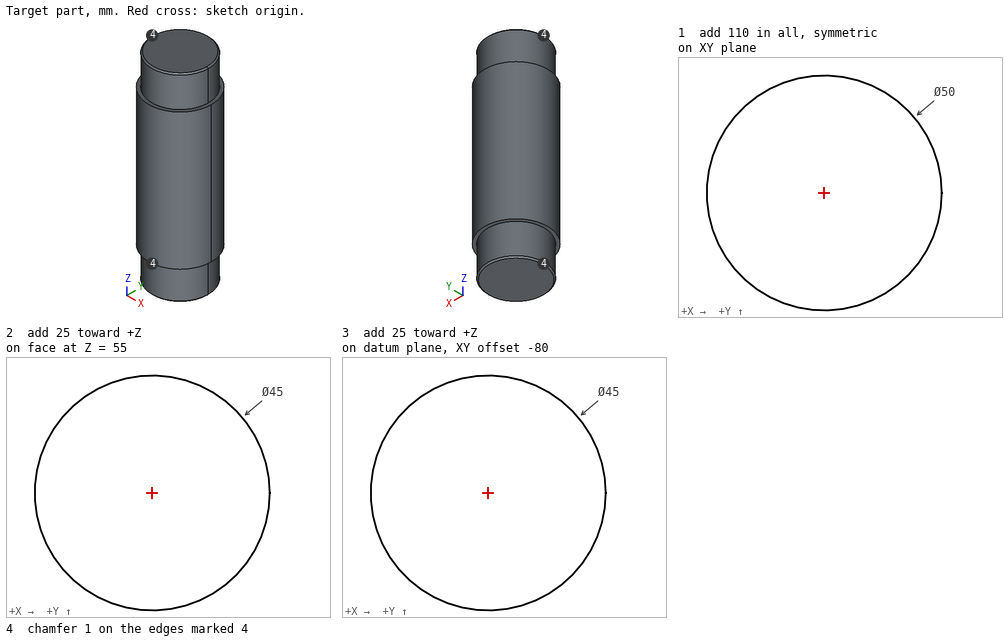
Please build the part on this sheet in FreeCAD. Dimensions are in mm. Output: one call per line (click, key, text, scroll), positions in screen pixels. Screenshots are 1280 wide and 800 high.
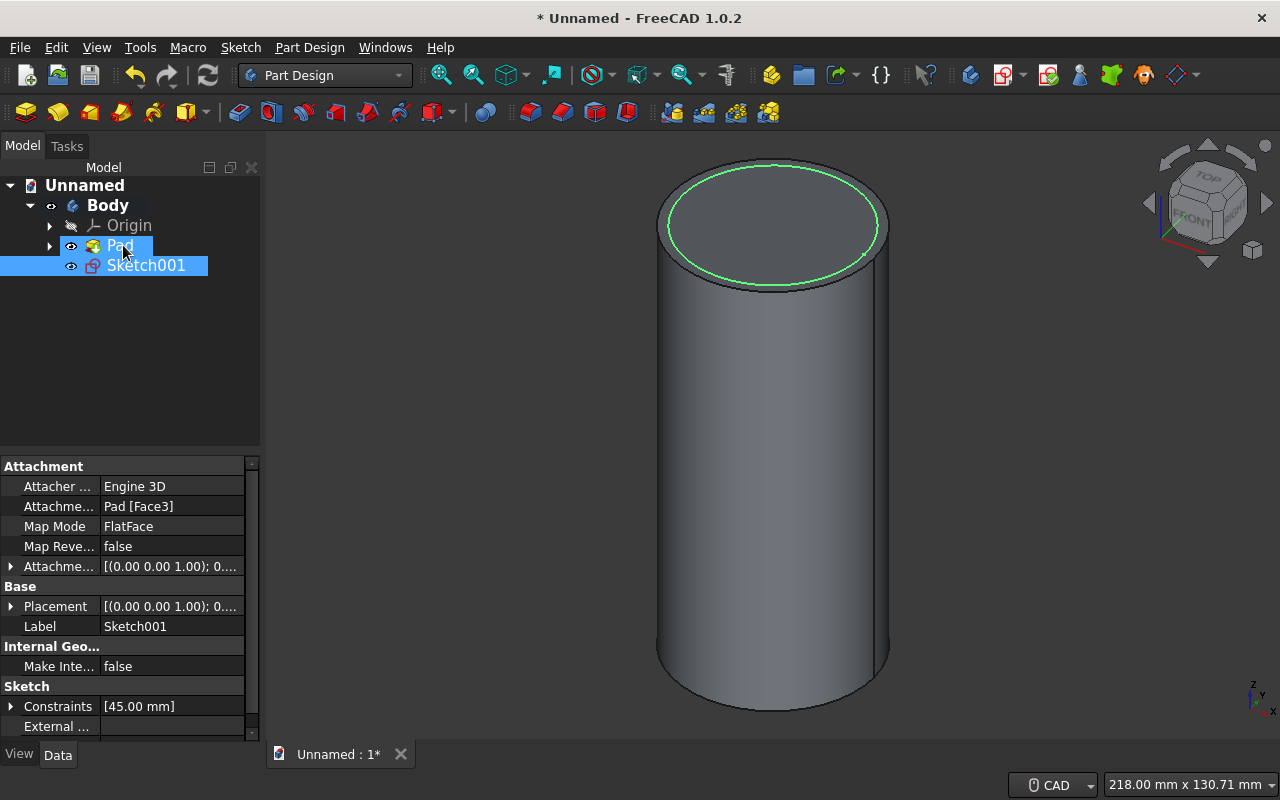
click(26, 112)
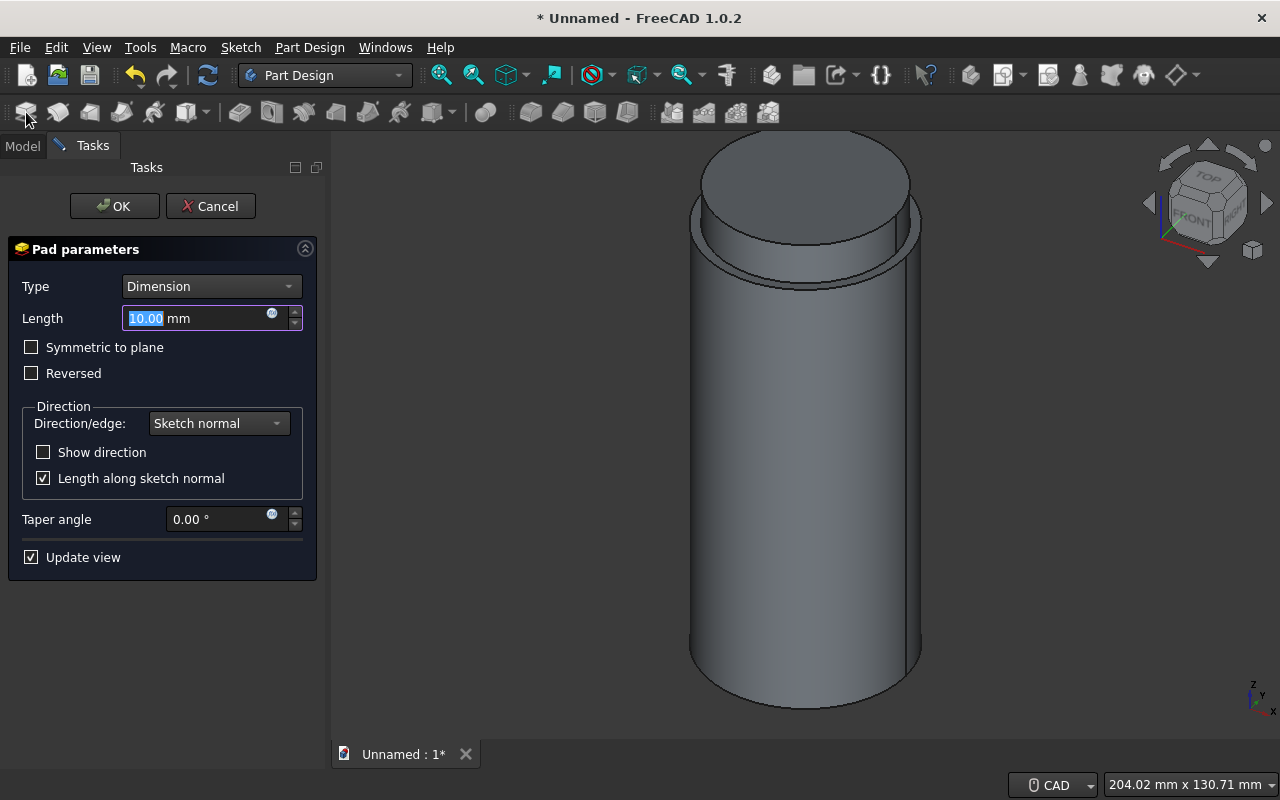
text(25)
key(Tab)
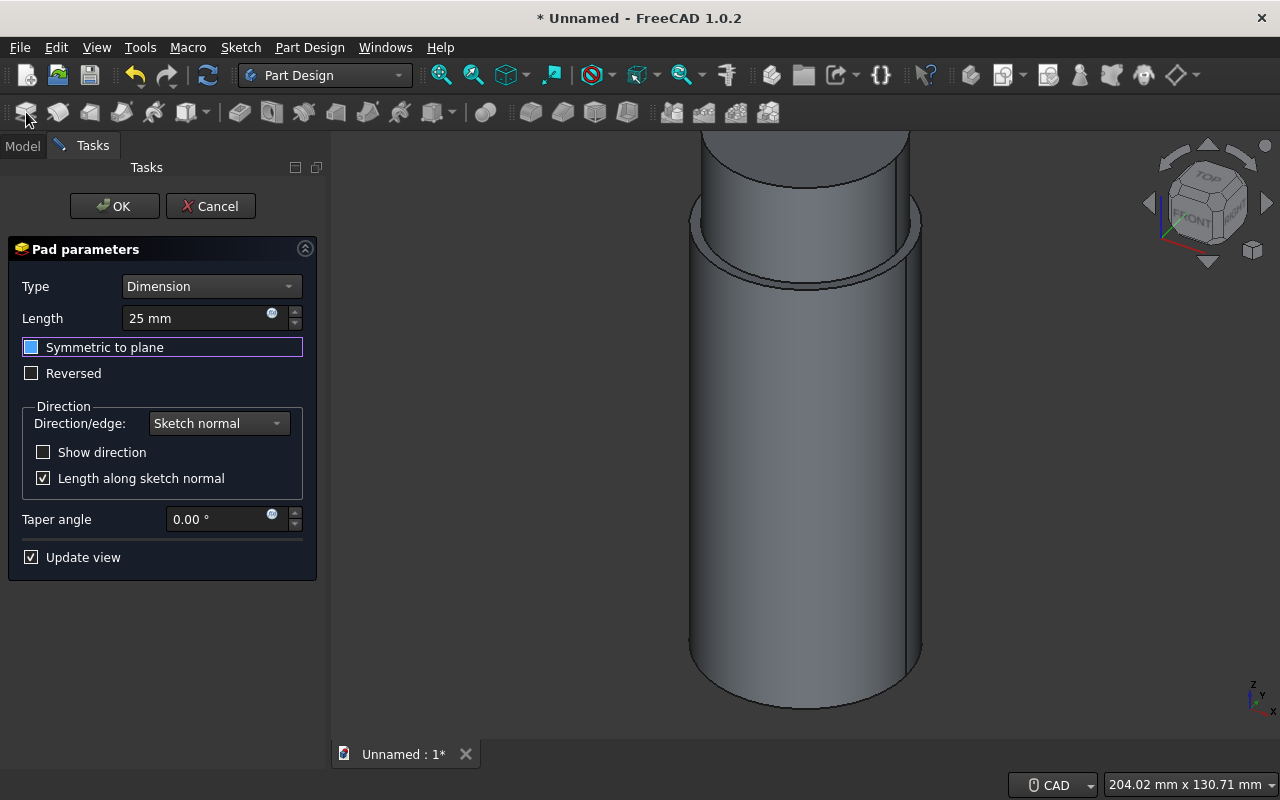
click(115, 206)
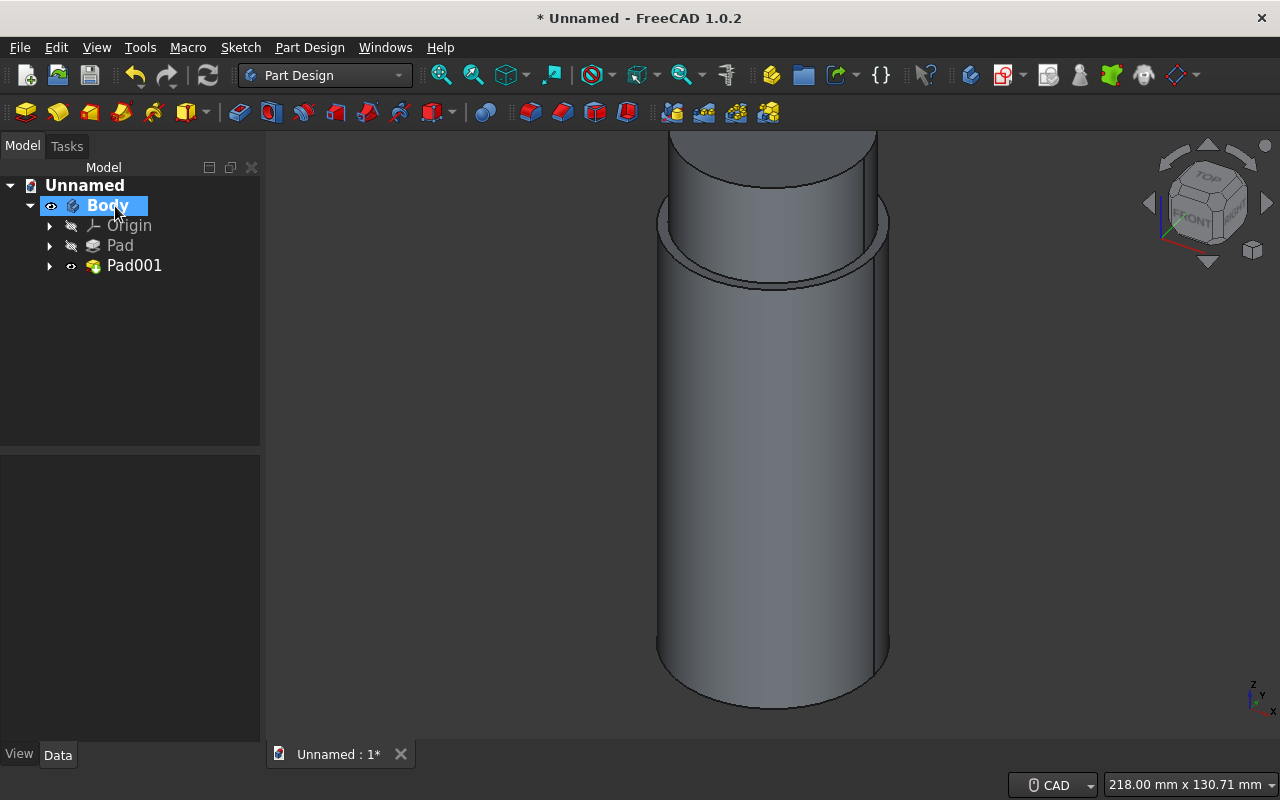
key(v)
key(f)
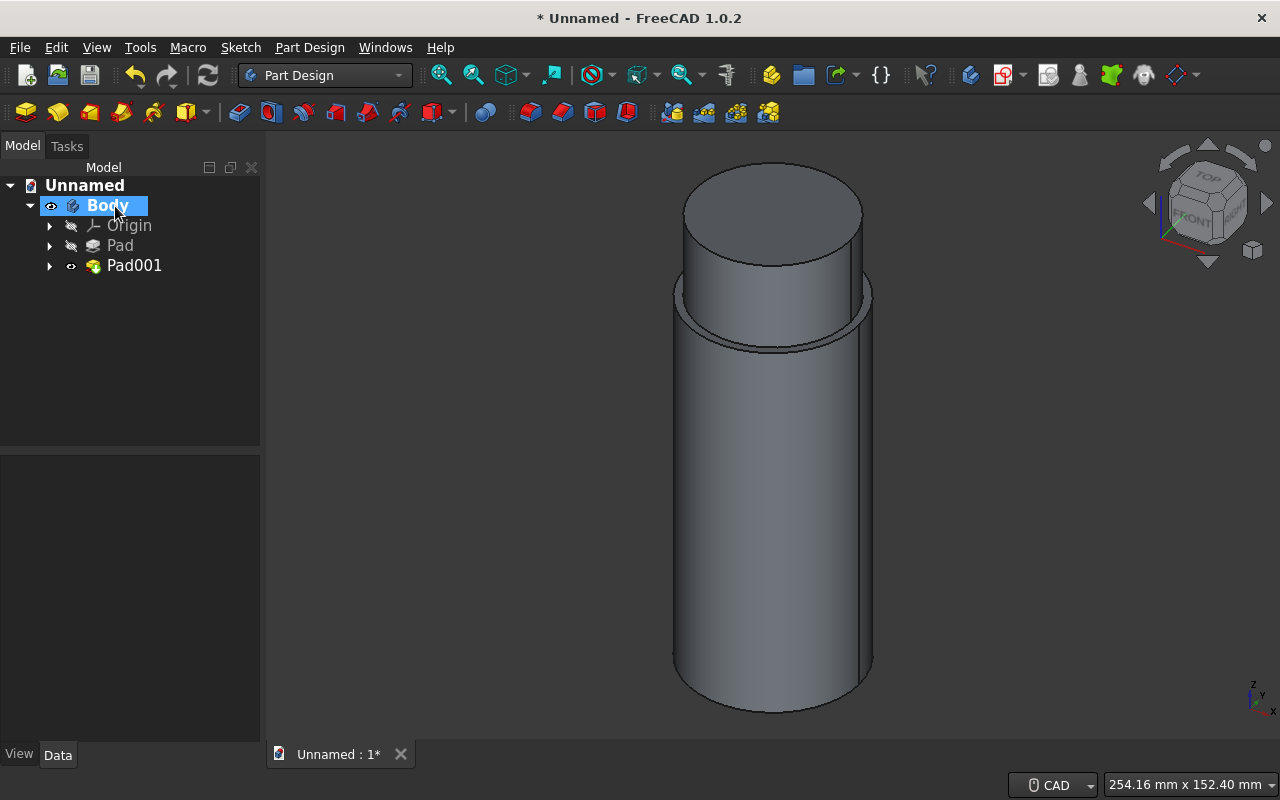
click(50, 226)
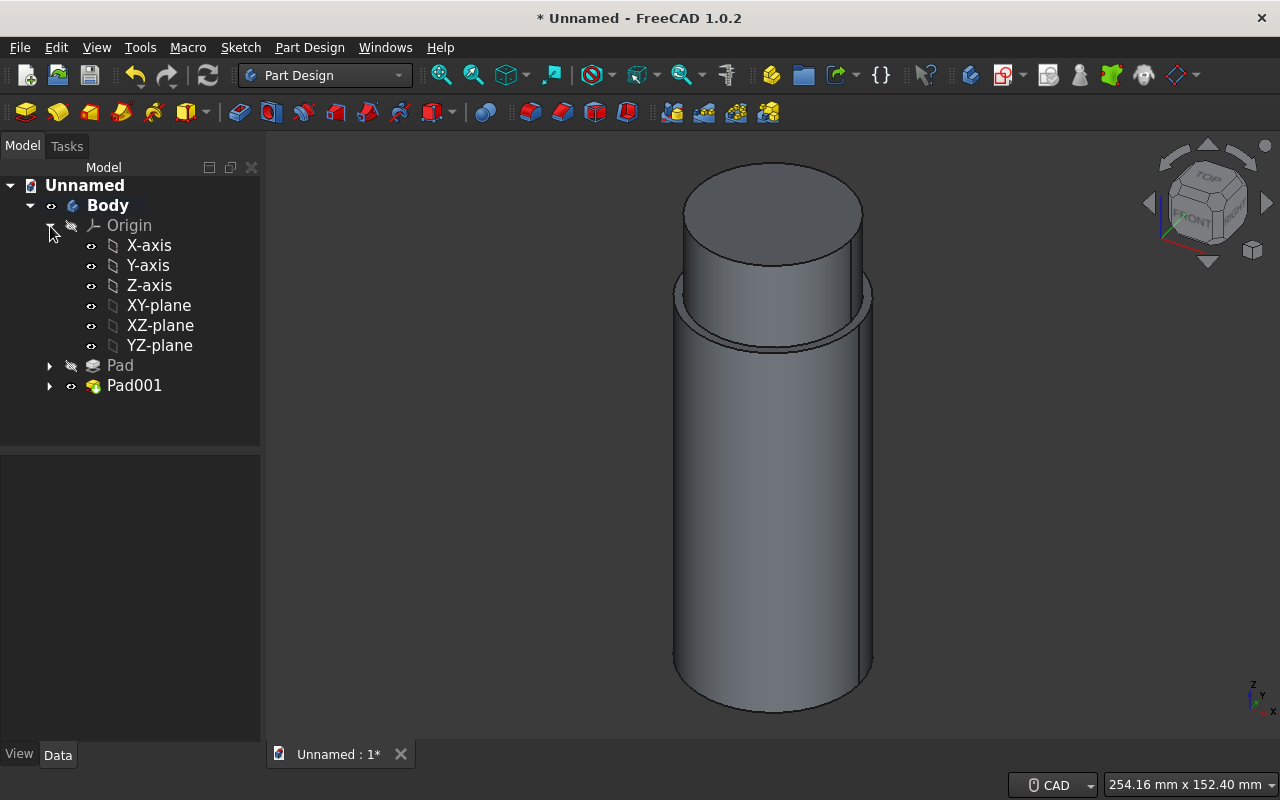
click(136, 306)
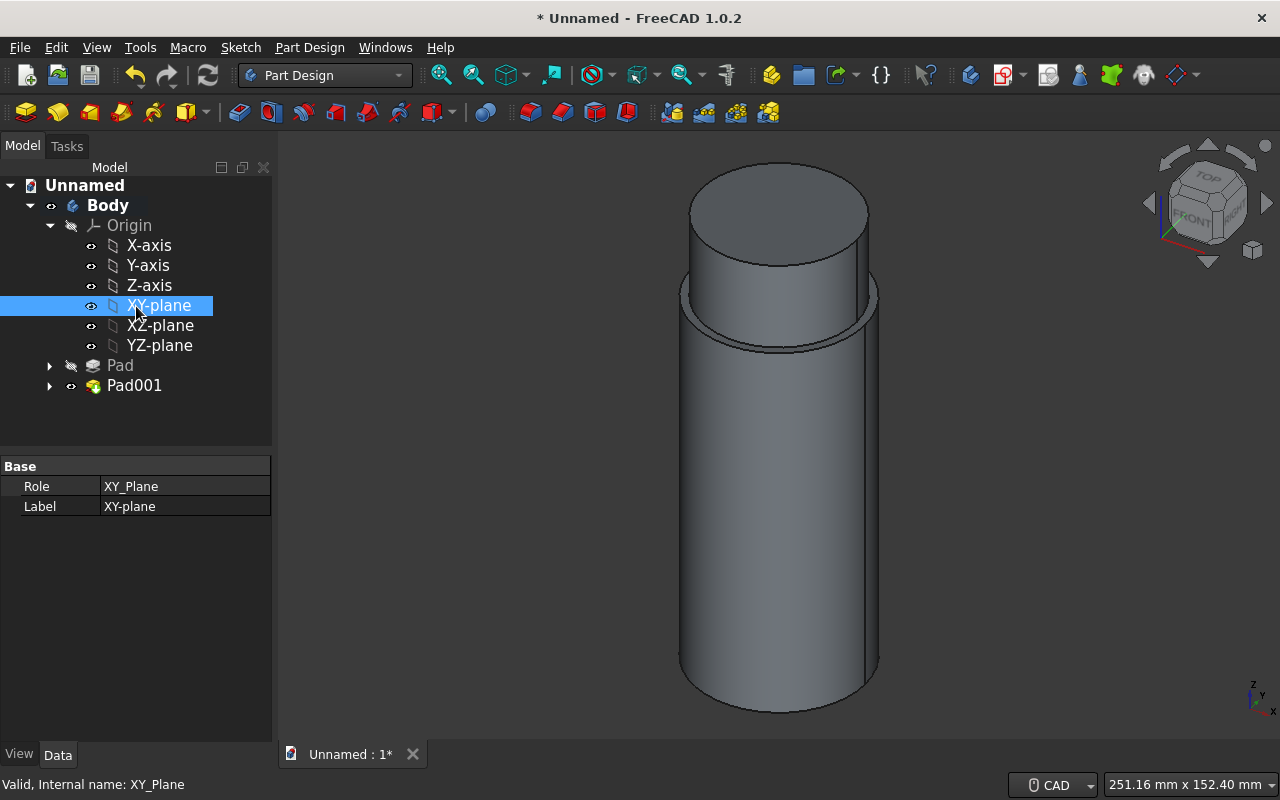
click(1176, 76)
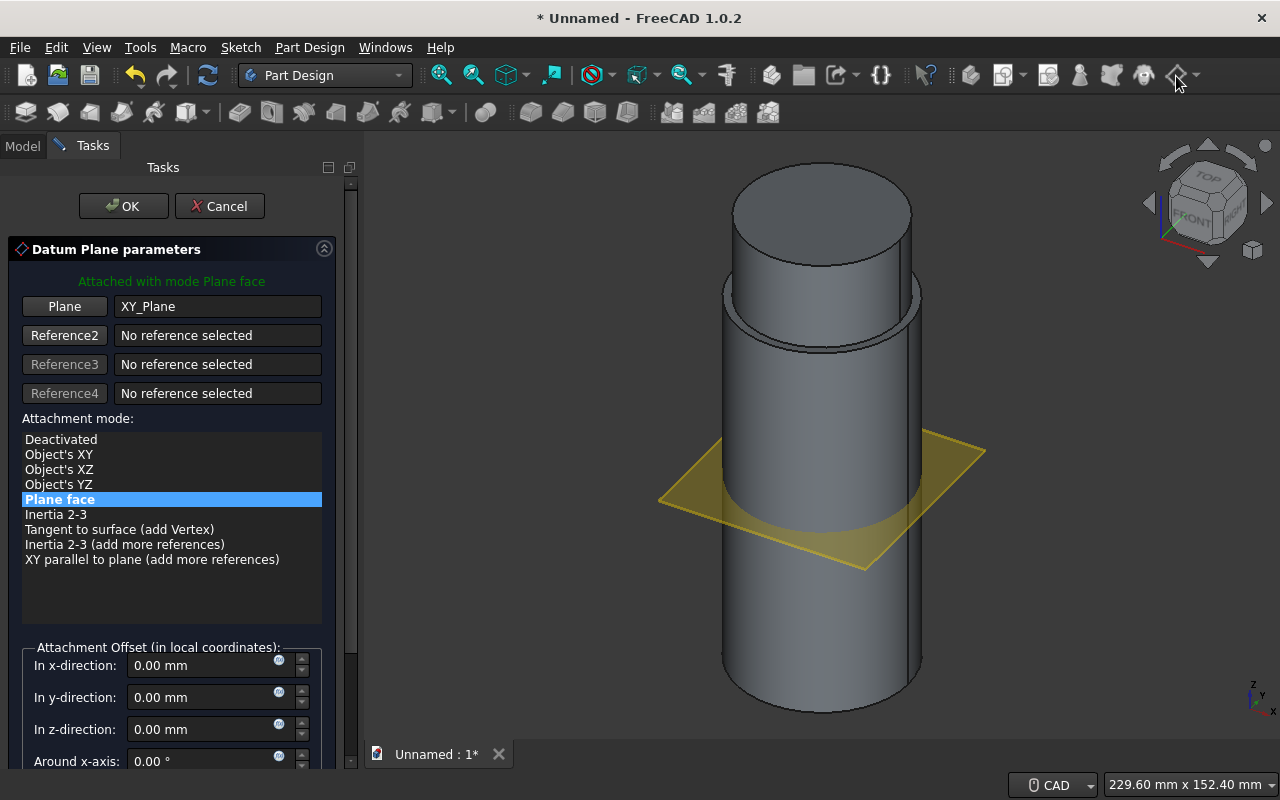
triple_click(210, 729)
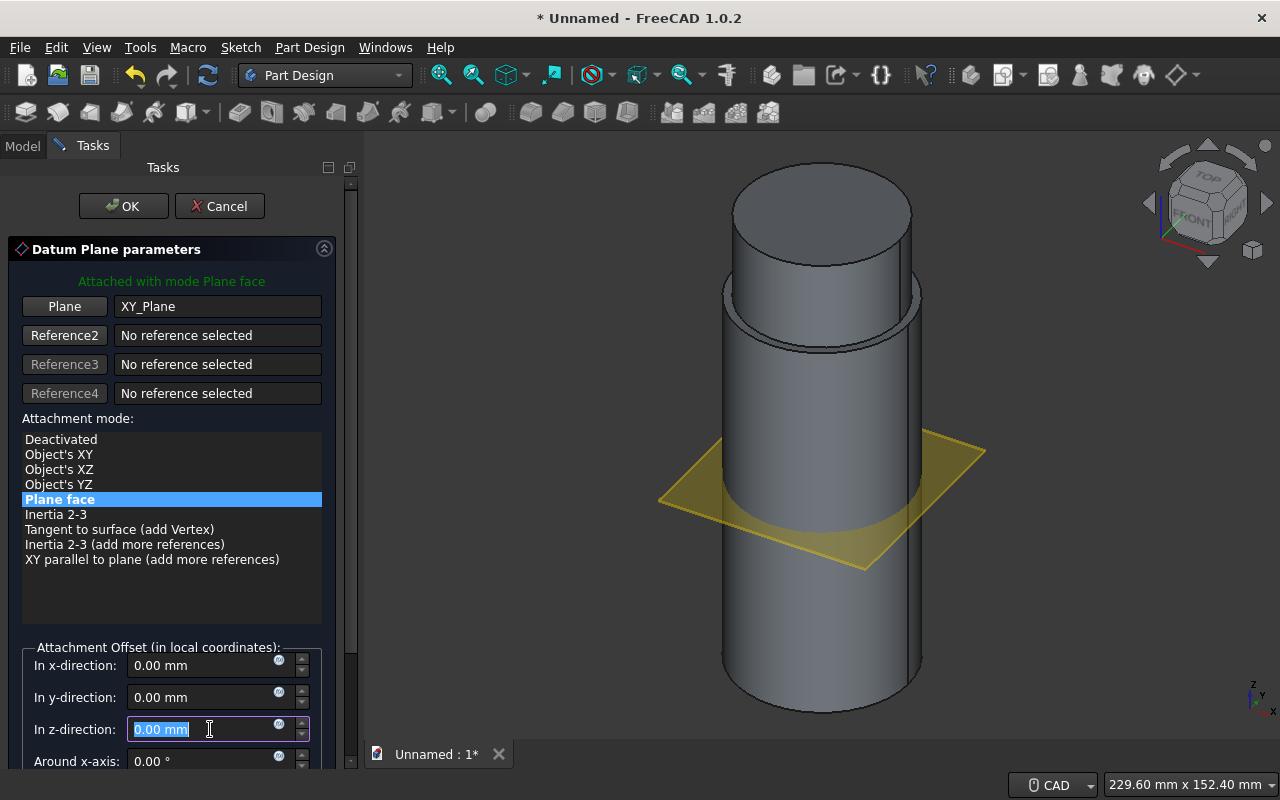
text(-80)
key(Tab)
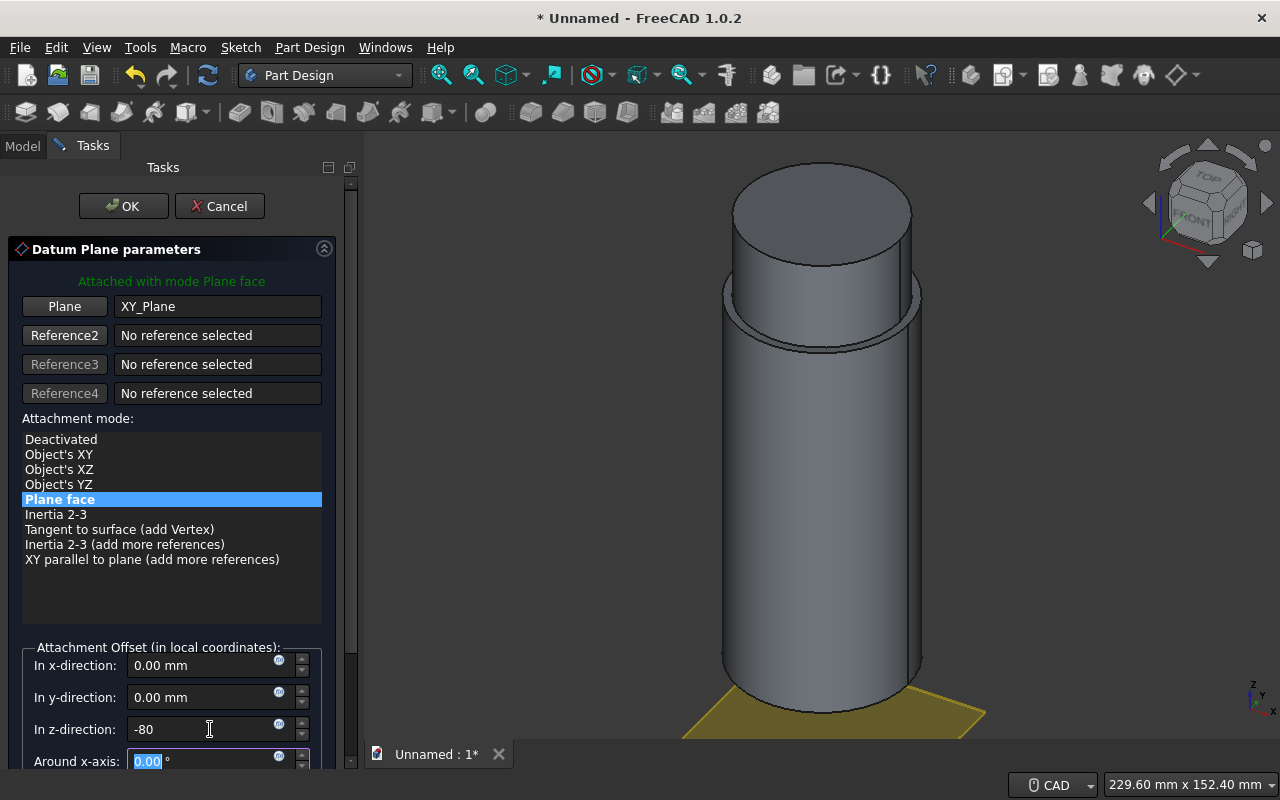
click(124, 206)